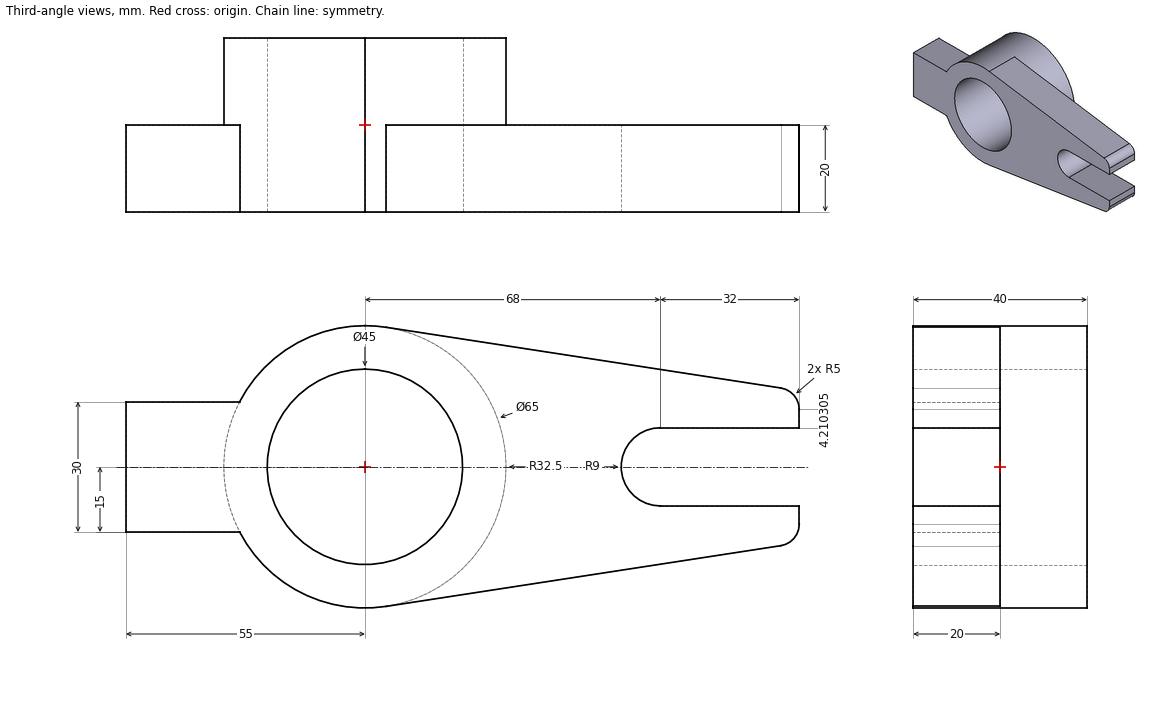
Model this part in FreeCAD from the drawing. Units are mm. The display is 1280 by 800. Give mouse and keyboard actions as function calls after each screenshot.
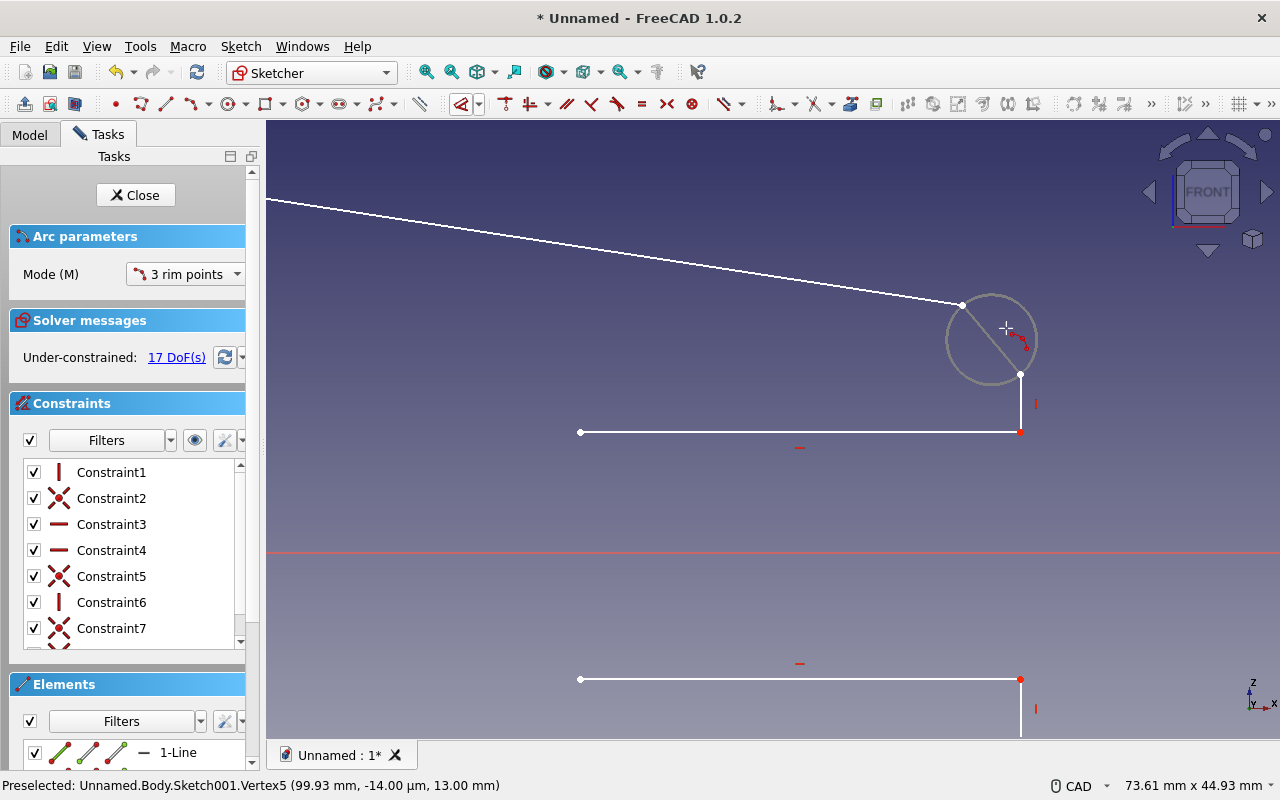
click(1005, 327)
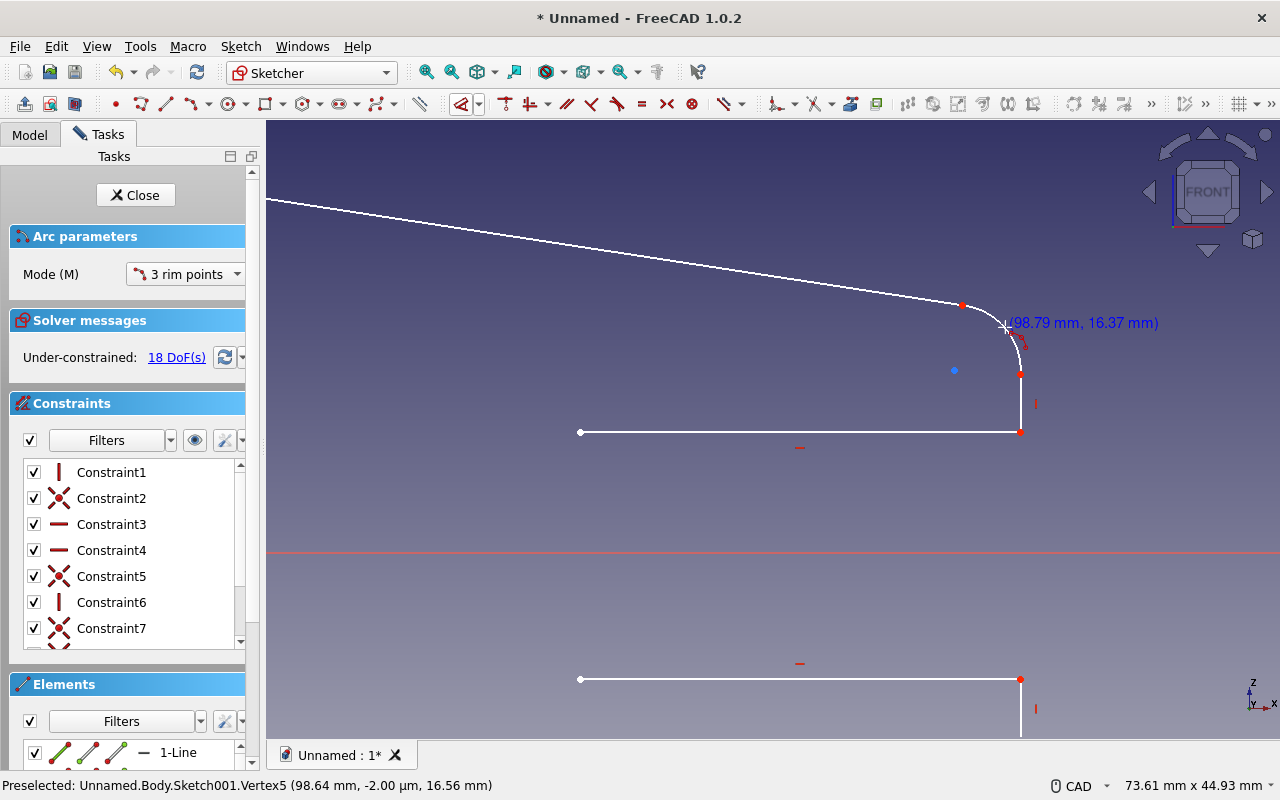
click(580, 432)
click(580, 679)
click(463, 515)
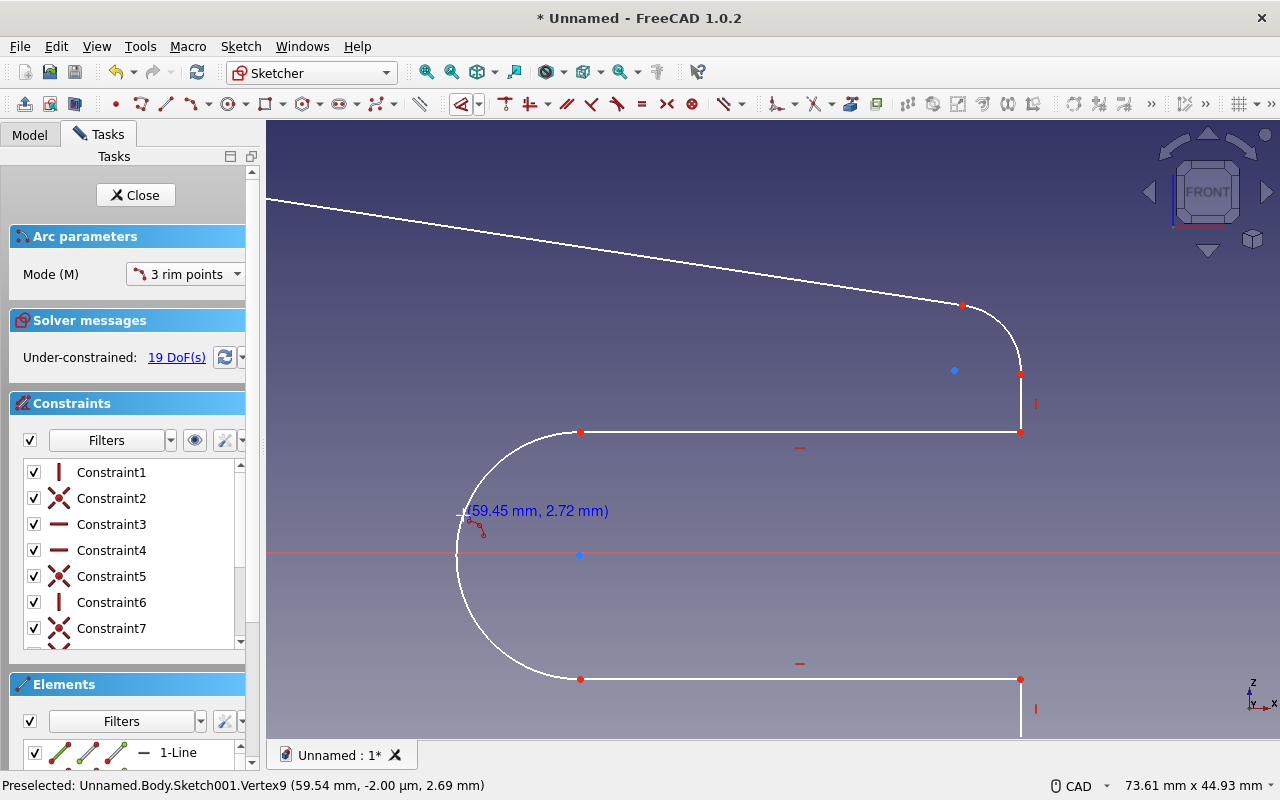
scroll(1008, 328, down, 4)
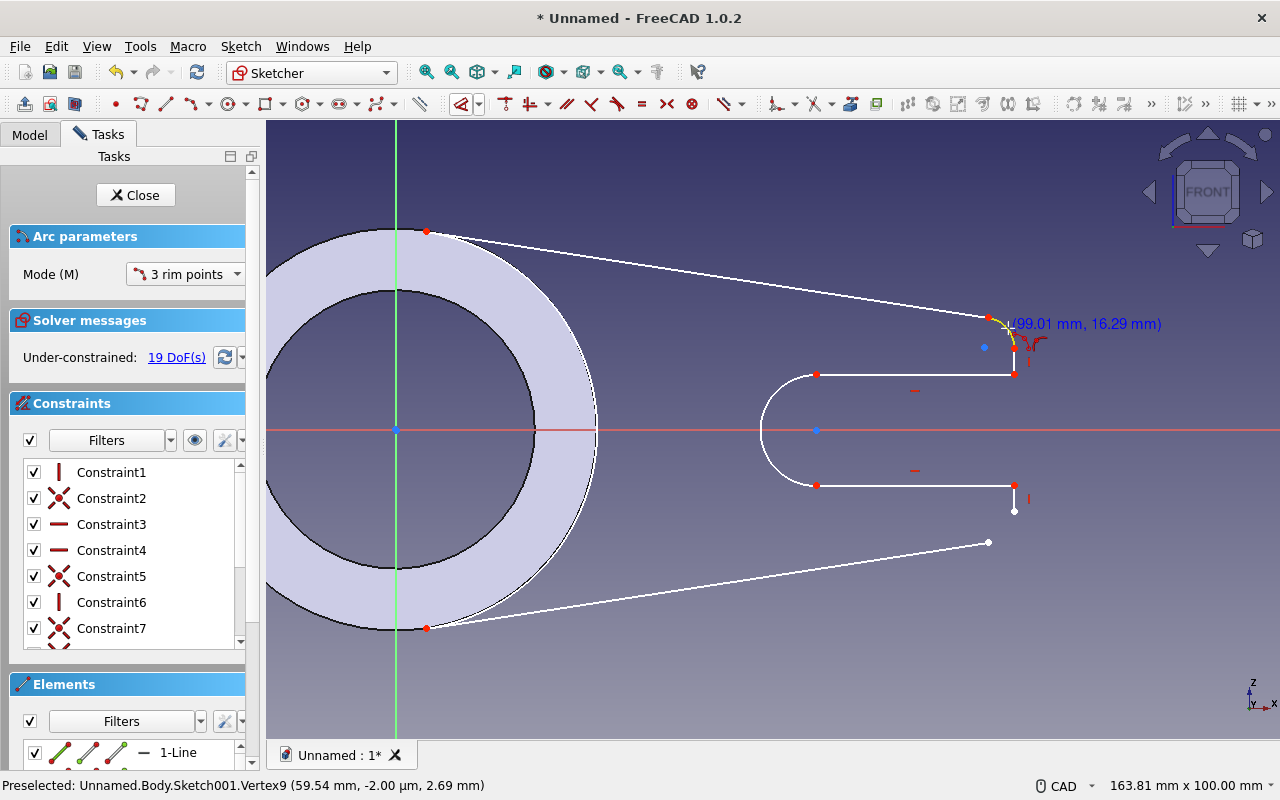
click(1014, 512)
click(988, 543)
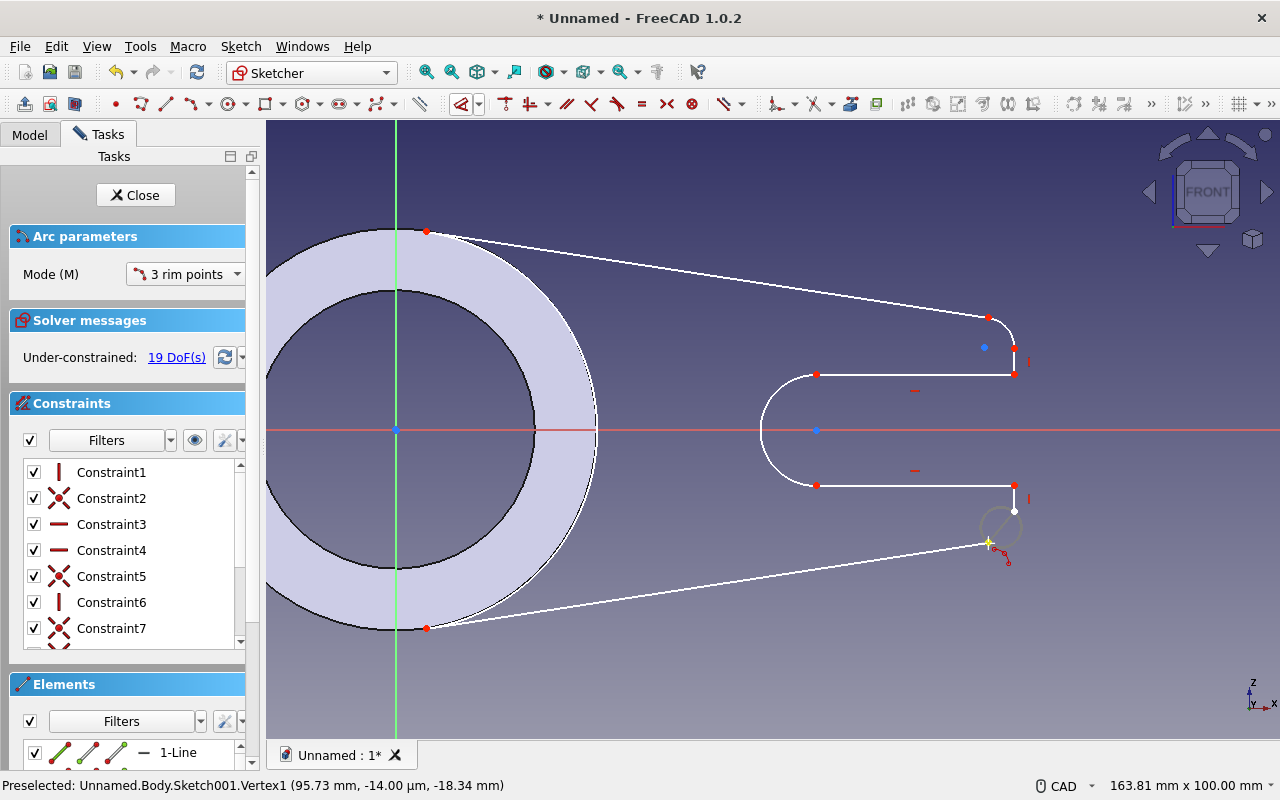
scroll(1007, 531, up, 4)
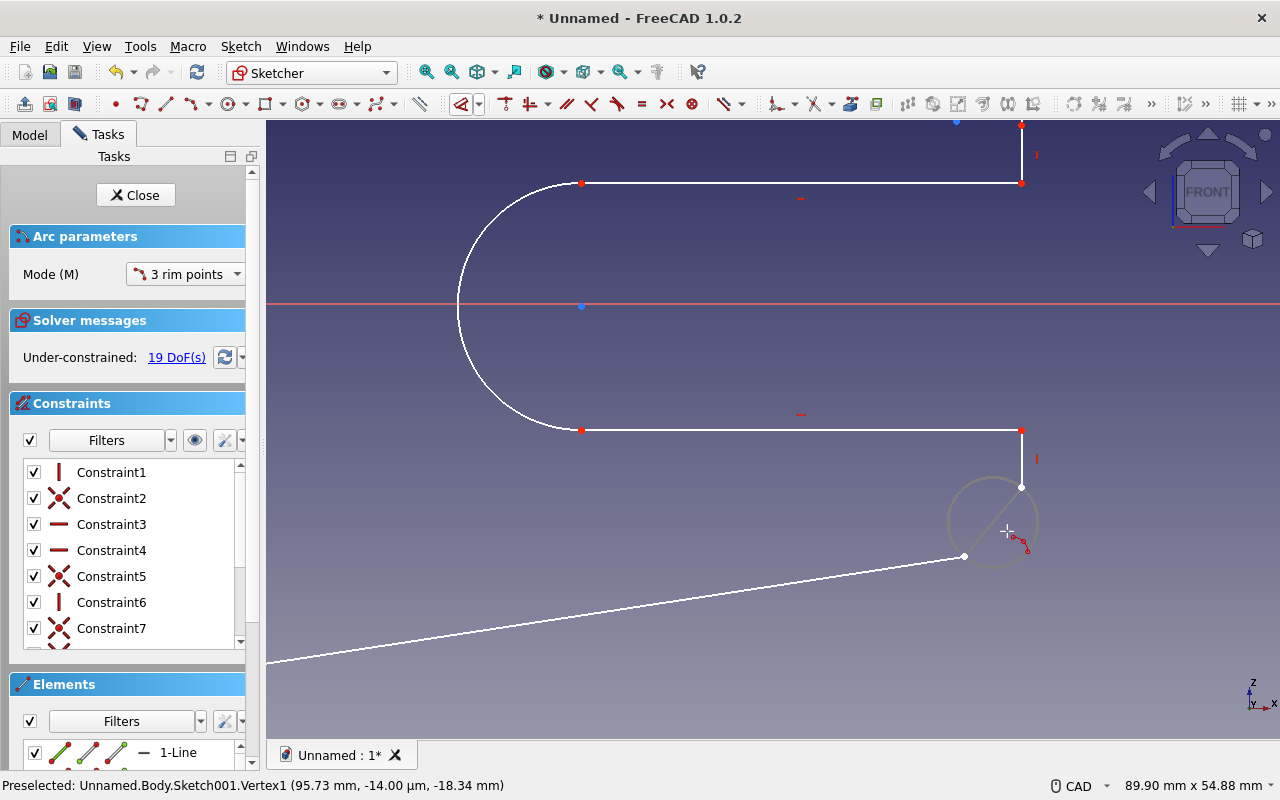
click(1006, 531)
key(Escape)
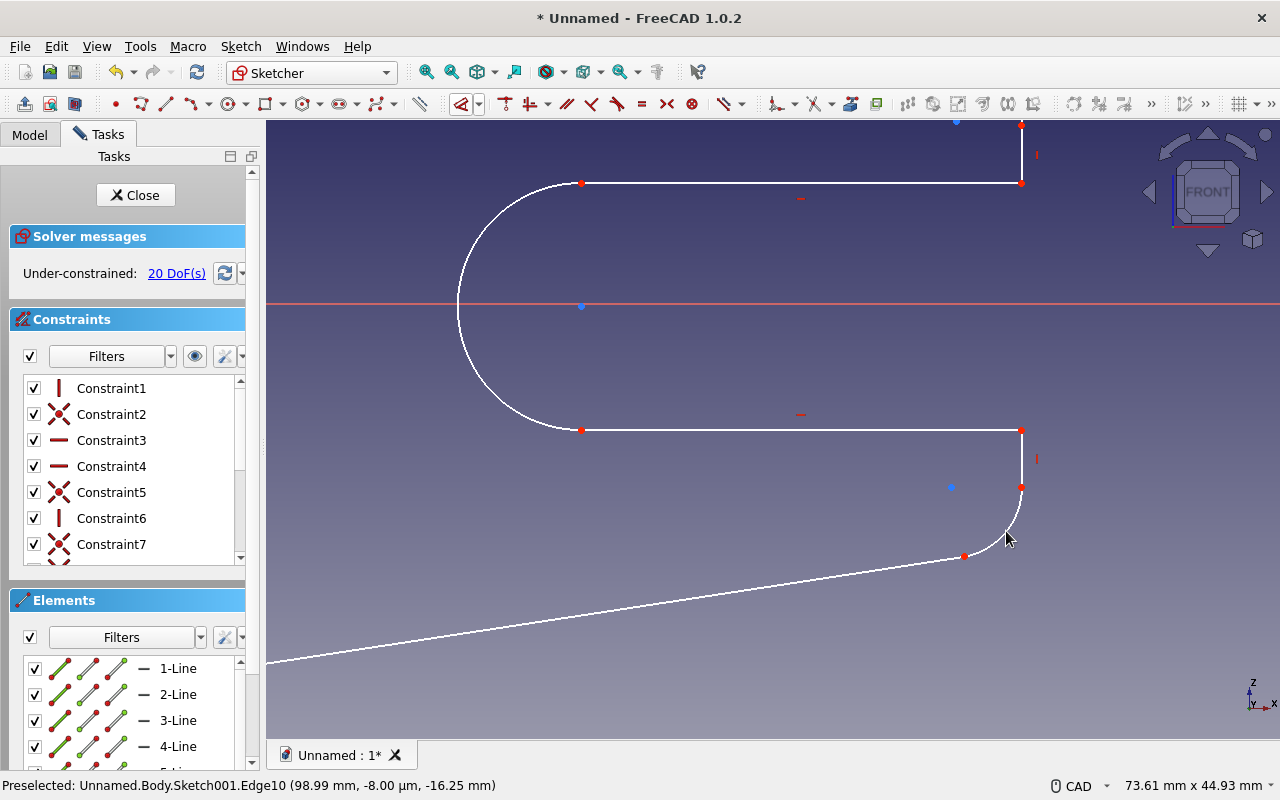
click(589, 614)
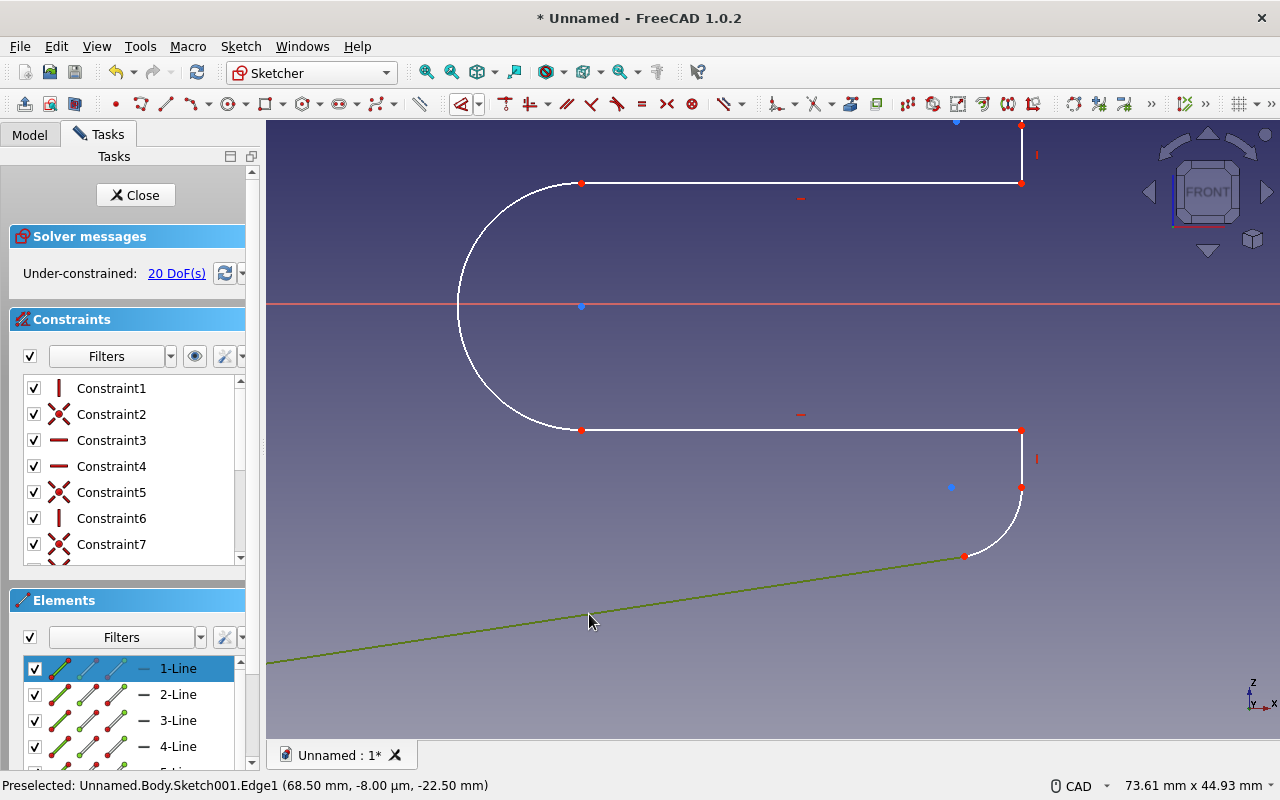
scroll(1007, 532, down, 4)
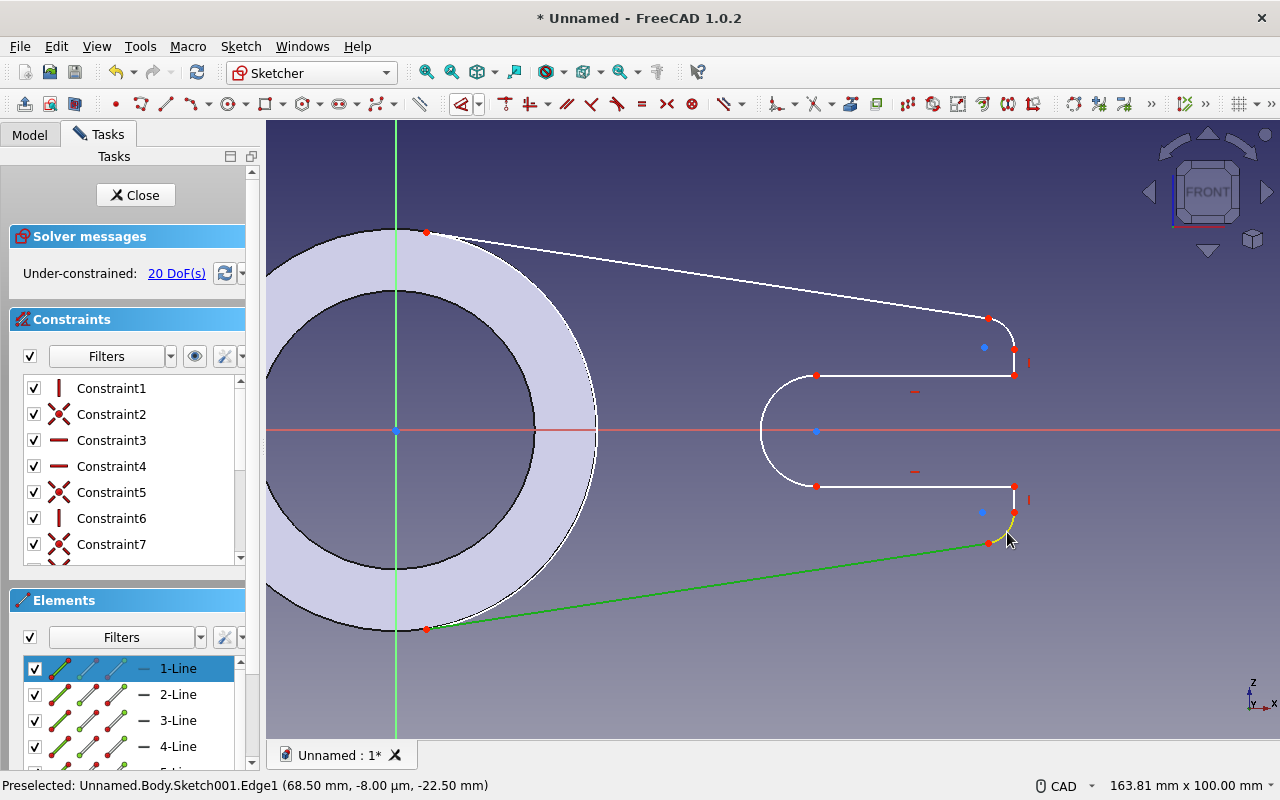
click(566, 539)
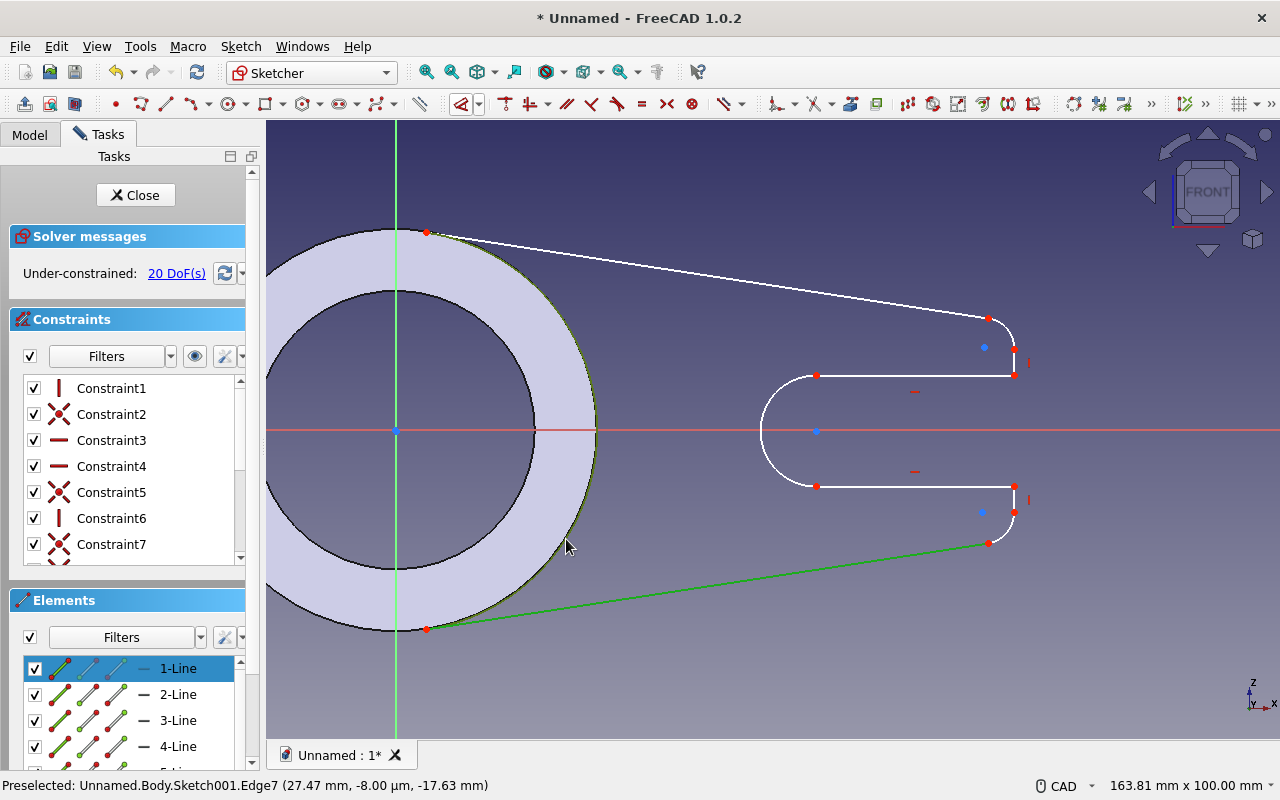
key(t)